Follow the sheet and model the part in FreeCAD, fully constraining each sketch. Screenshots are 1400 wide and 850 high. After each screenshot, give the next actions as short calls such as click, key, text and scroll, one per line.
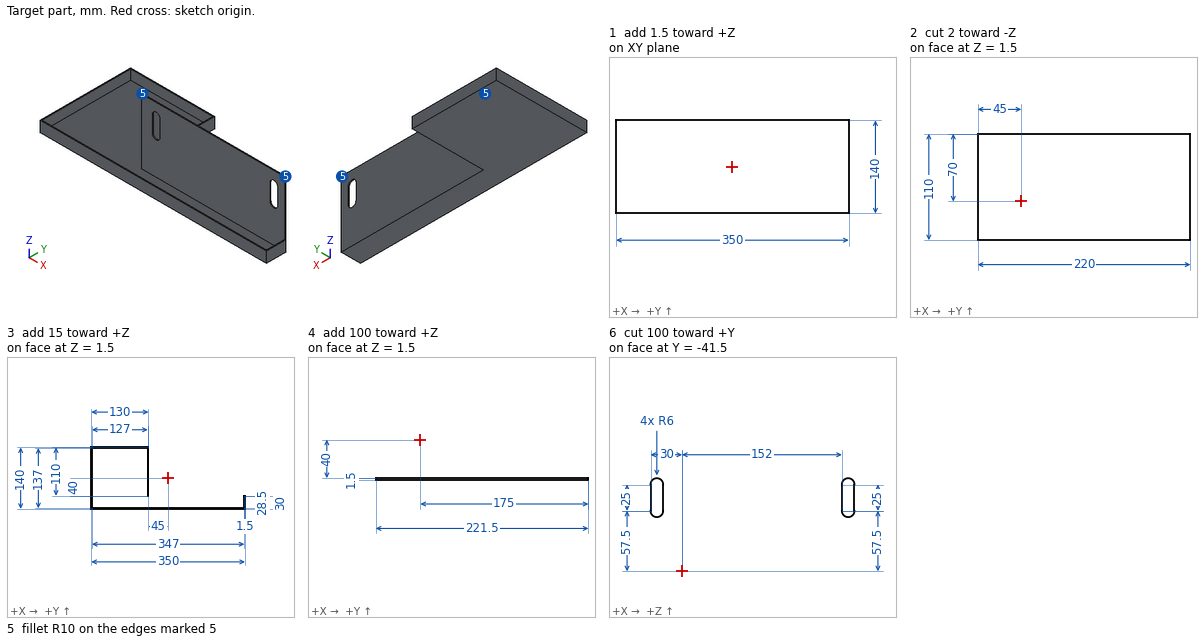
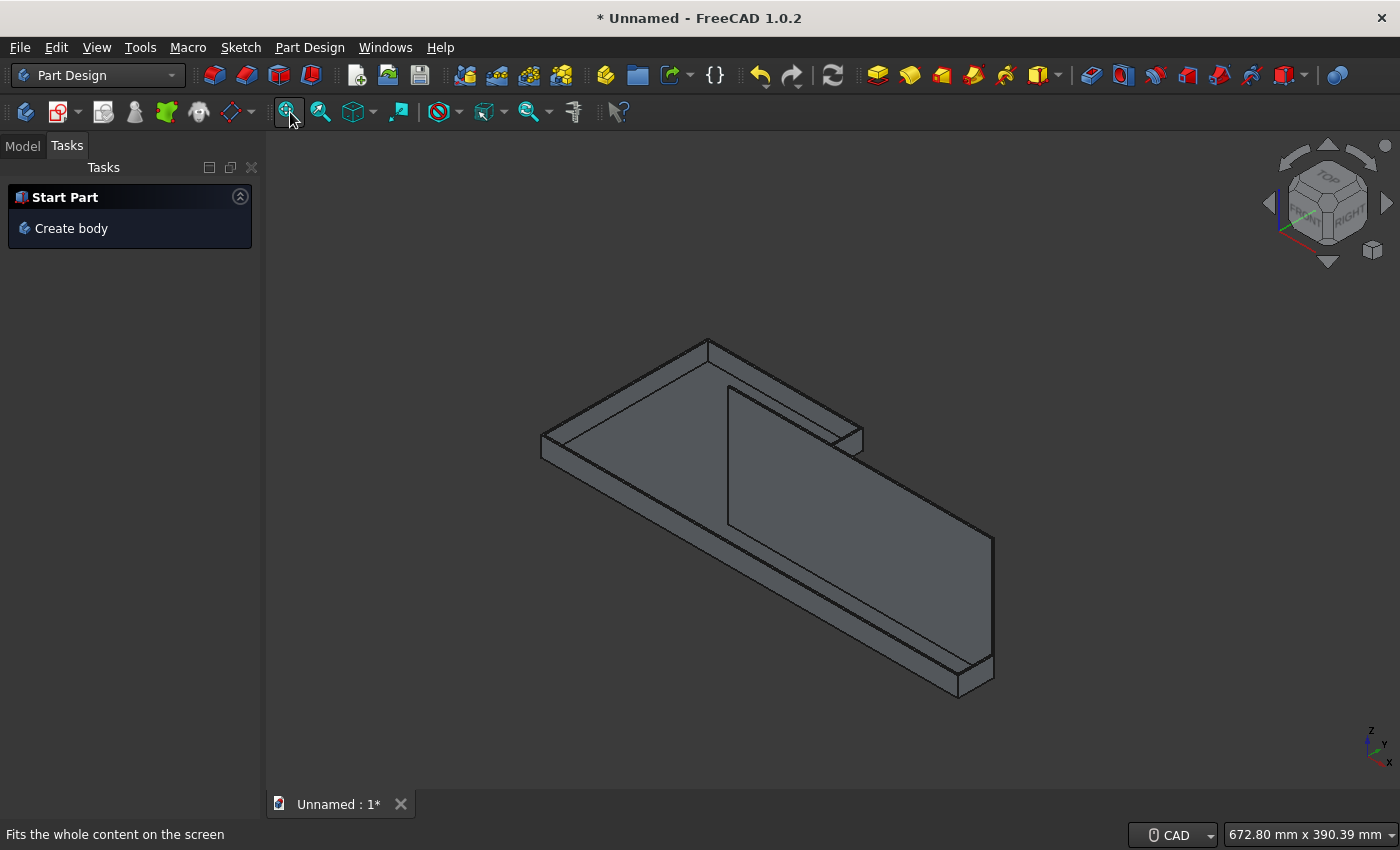
scroll(729, 385, up, 14)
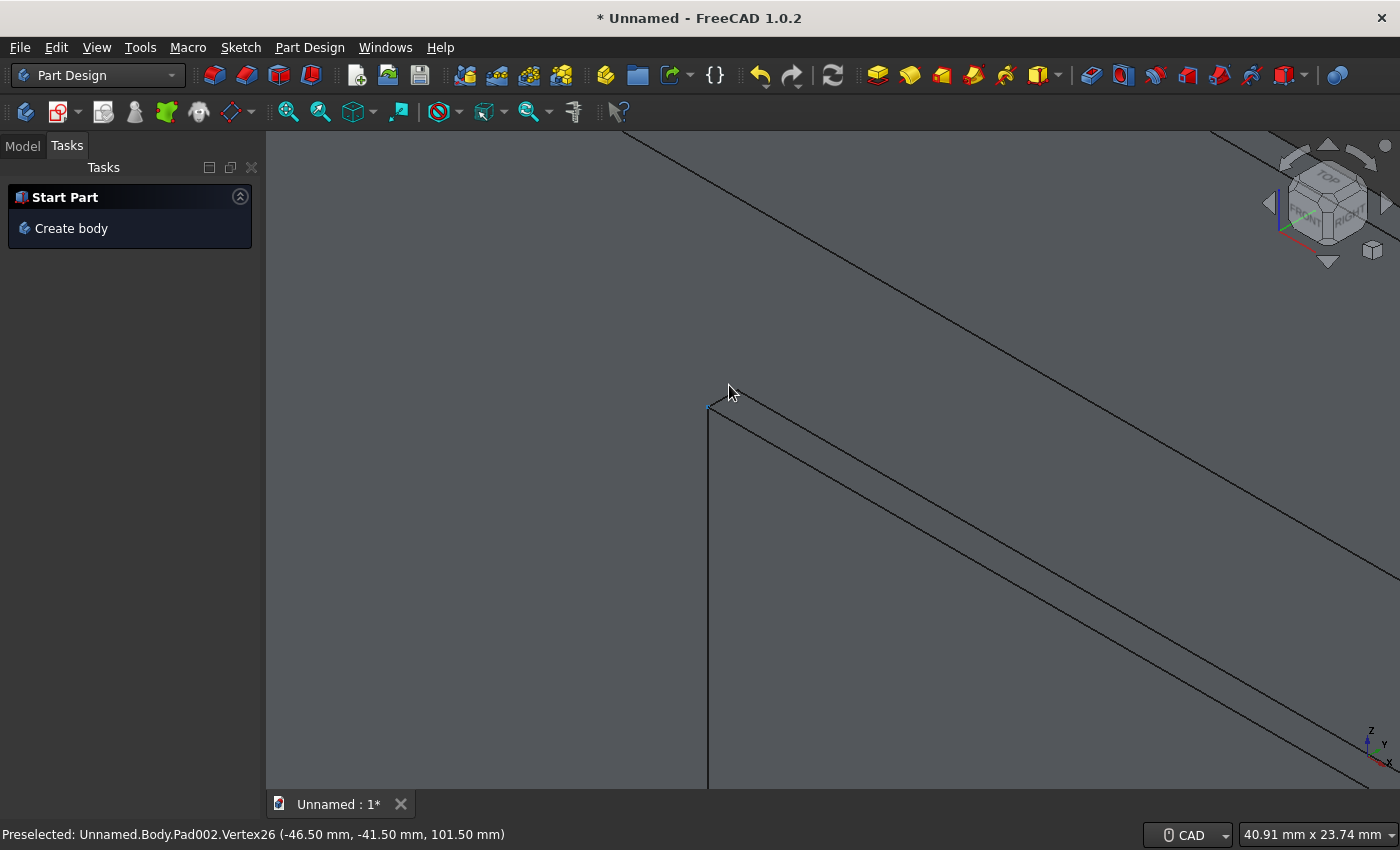
click(290, 112)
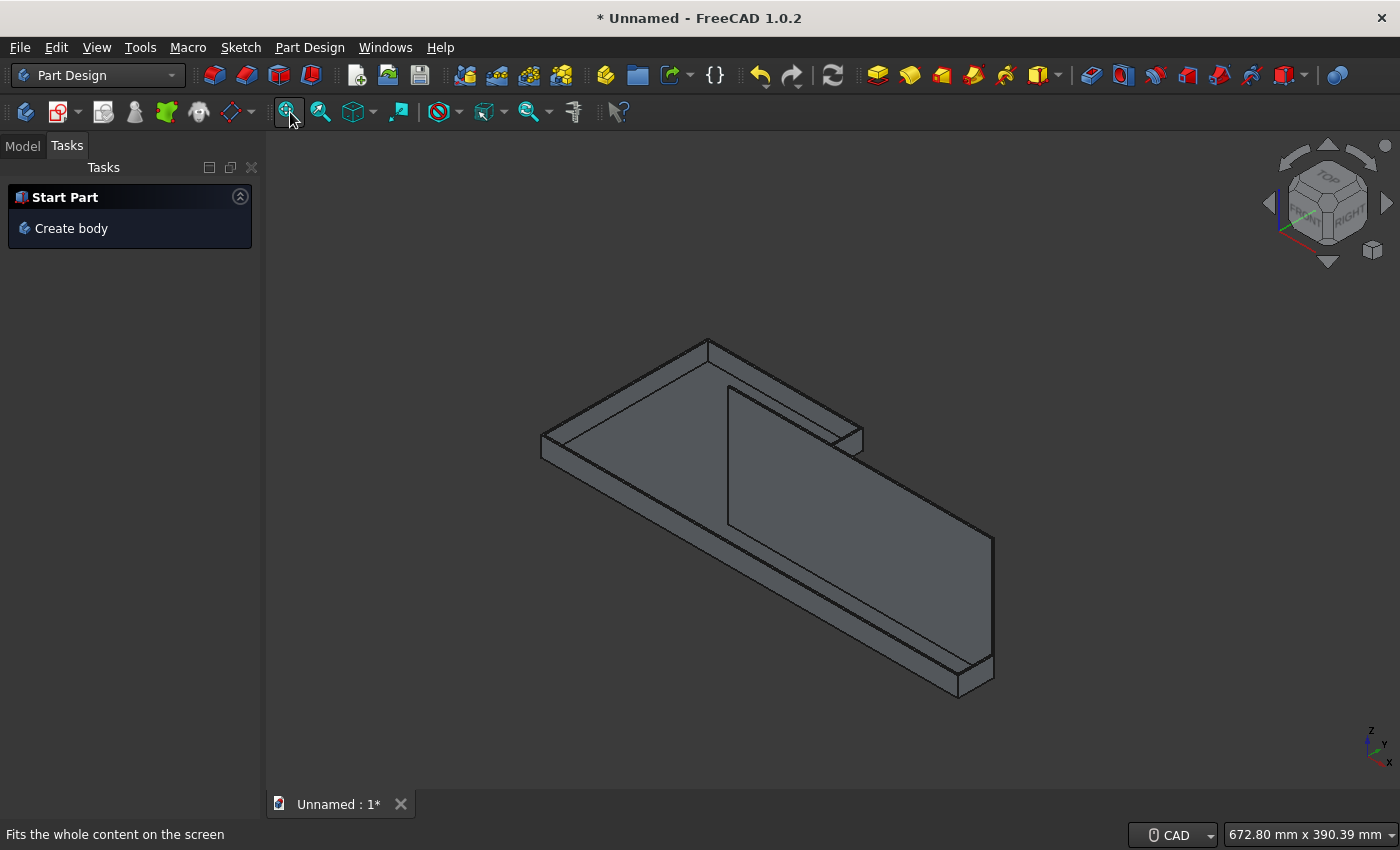
key(2)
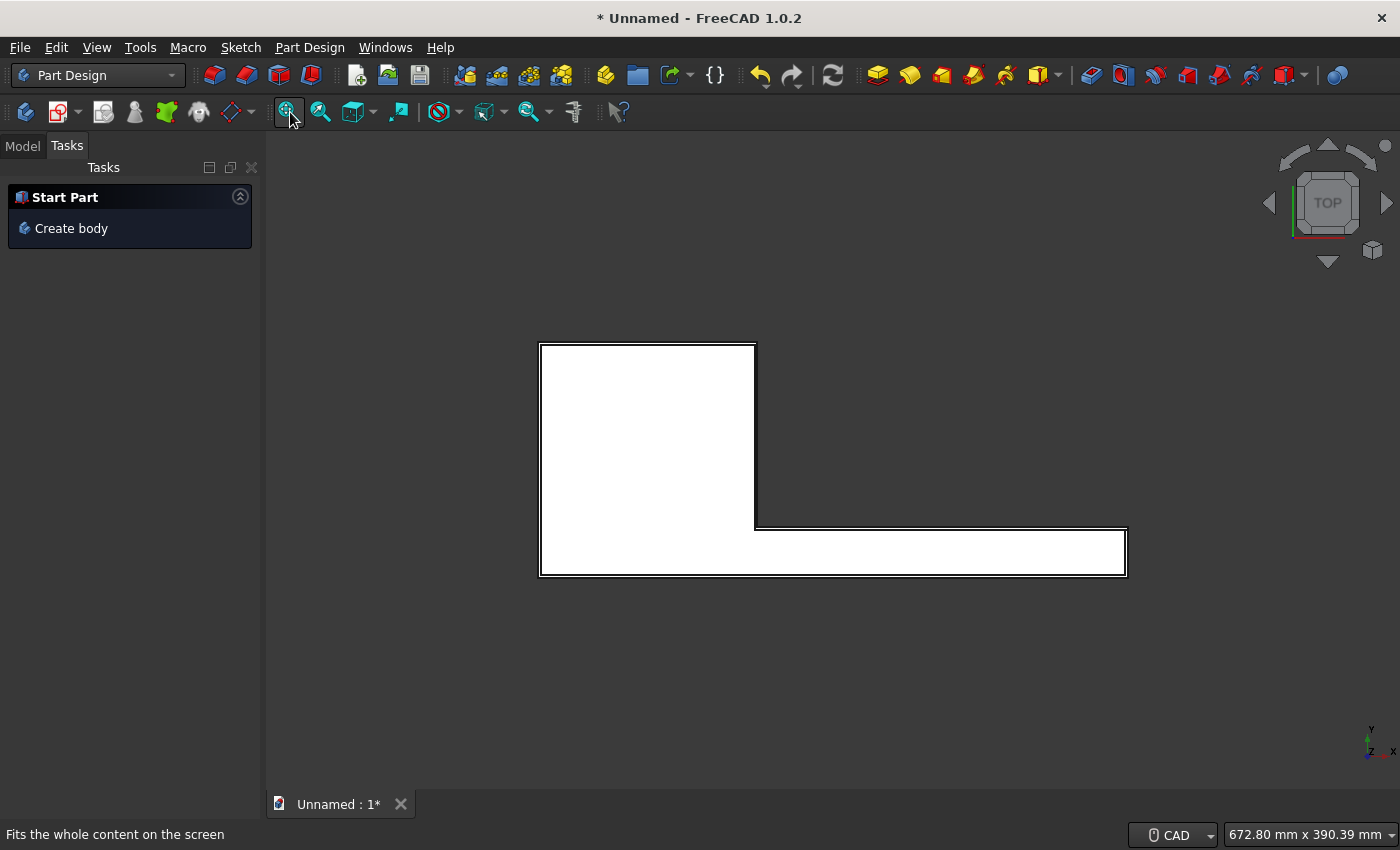
scroll(755, 528, up, 14)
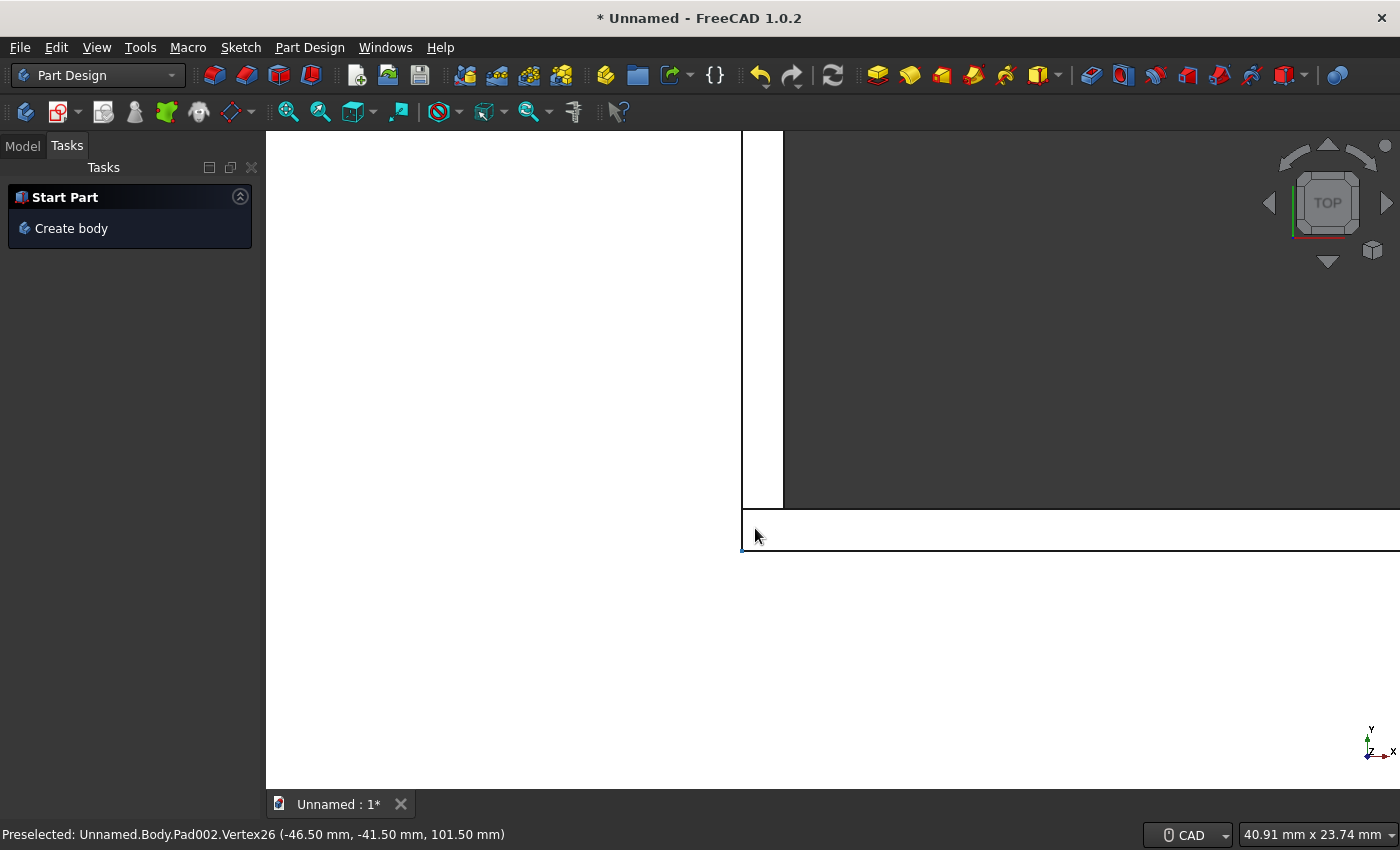
click(742, 529)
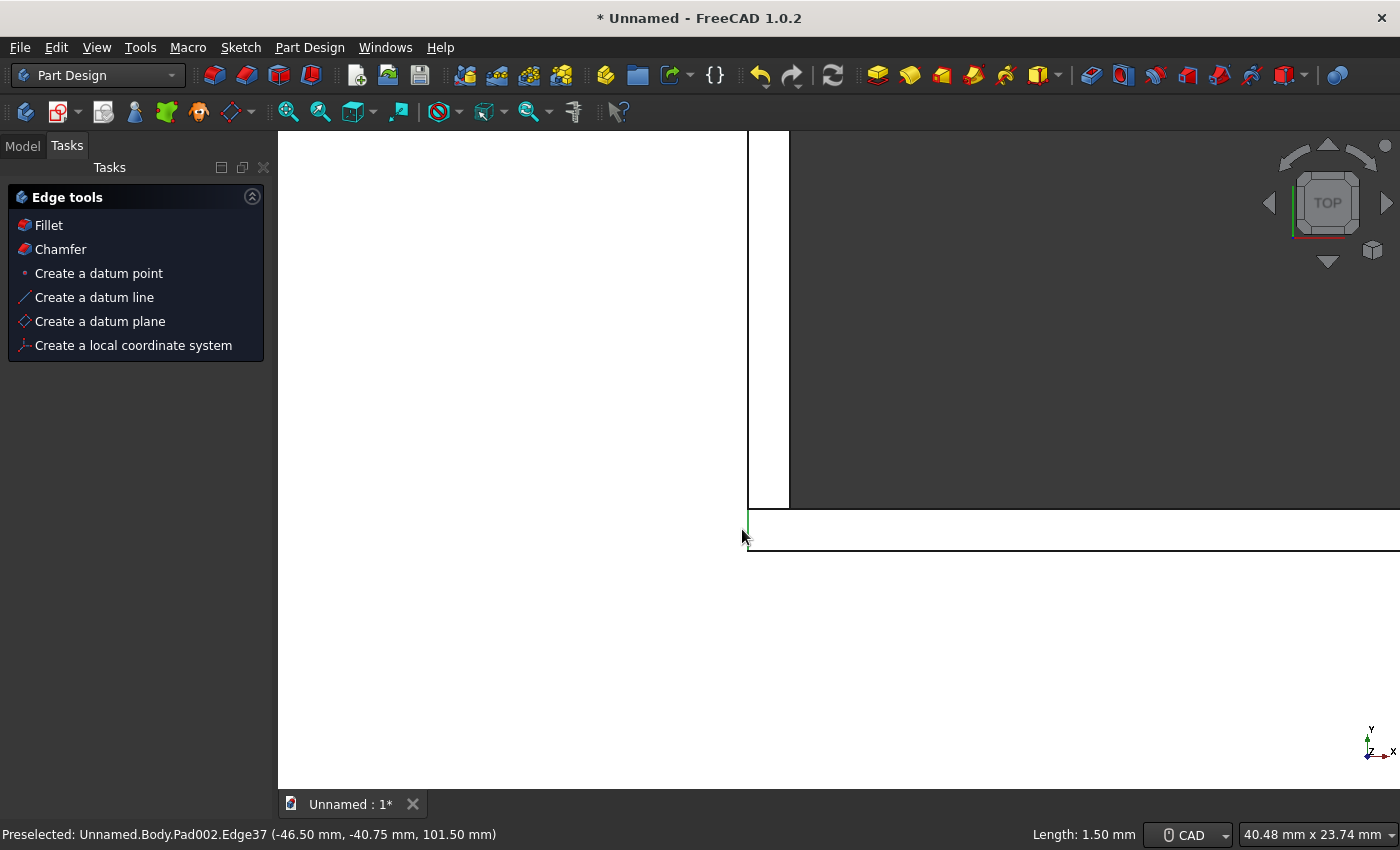
click(290, 112)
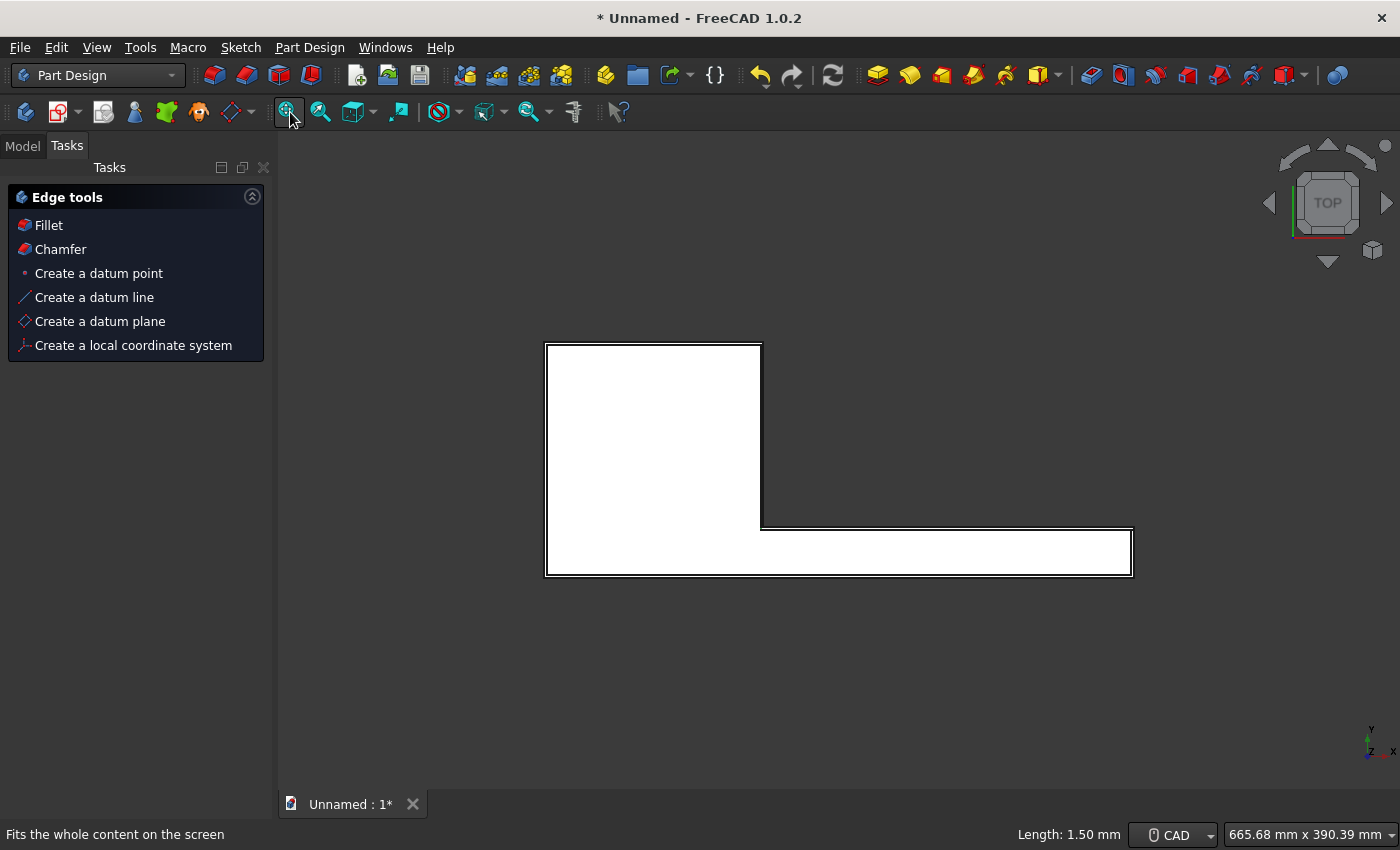
key(1)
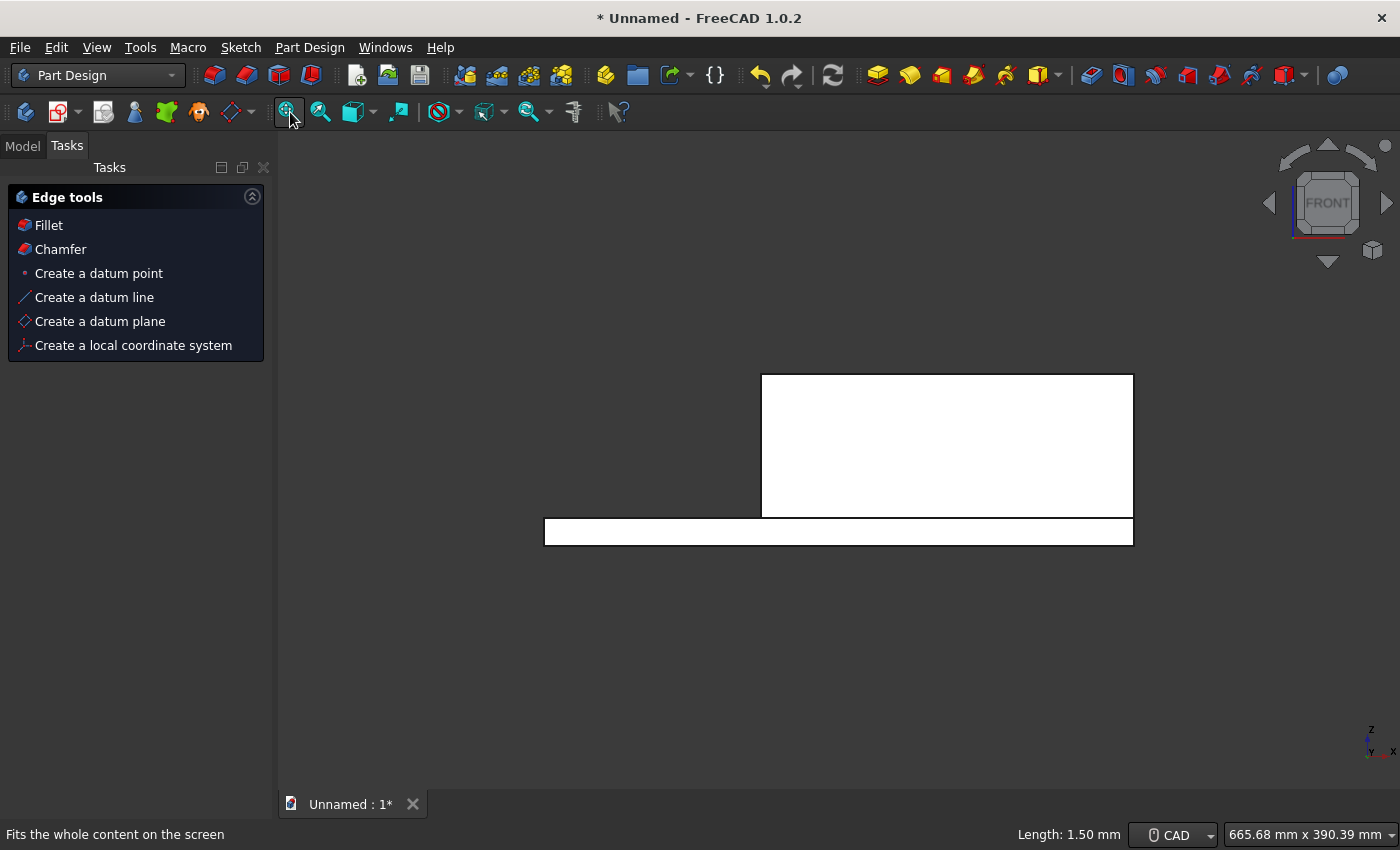
scroll(1134, 373, up, 14)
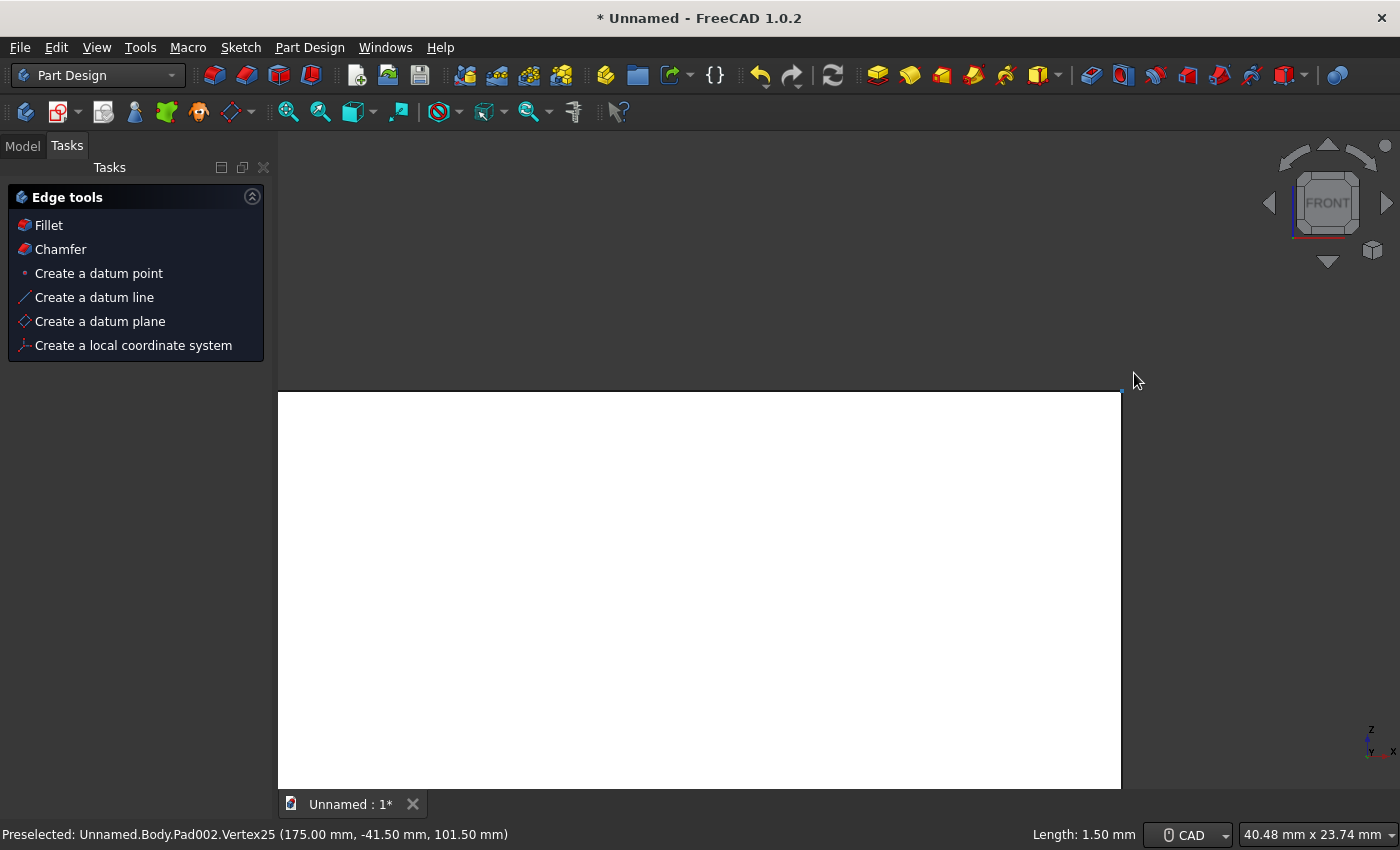
click(290, 112)